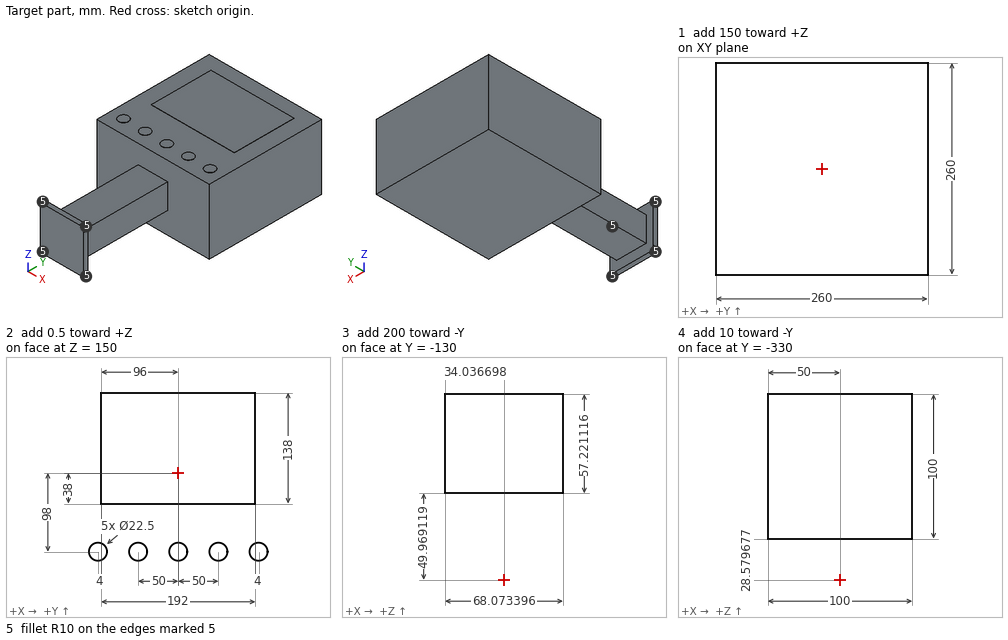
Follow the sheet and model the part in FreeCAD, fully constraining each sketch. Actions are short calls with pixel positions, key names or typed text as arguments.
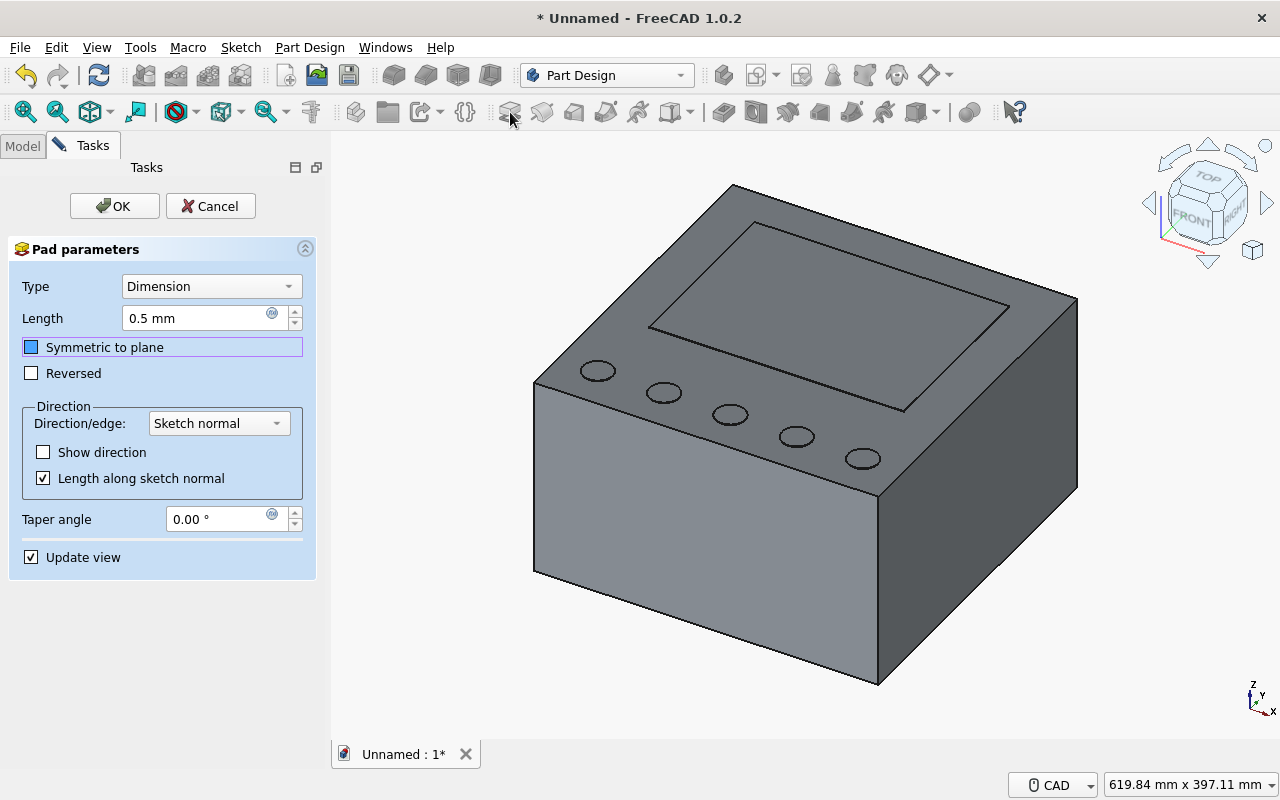
click(115, 206)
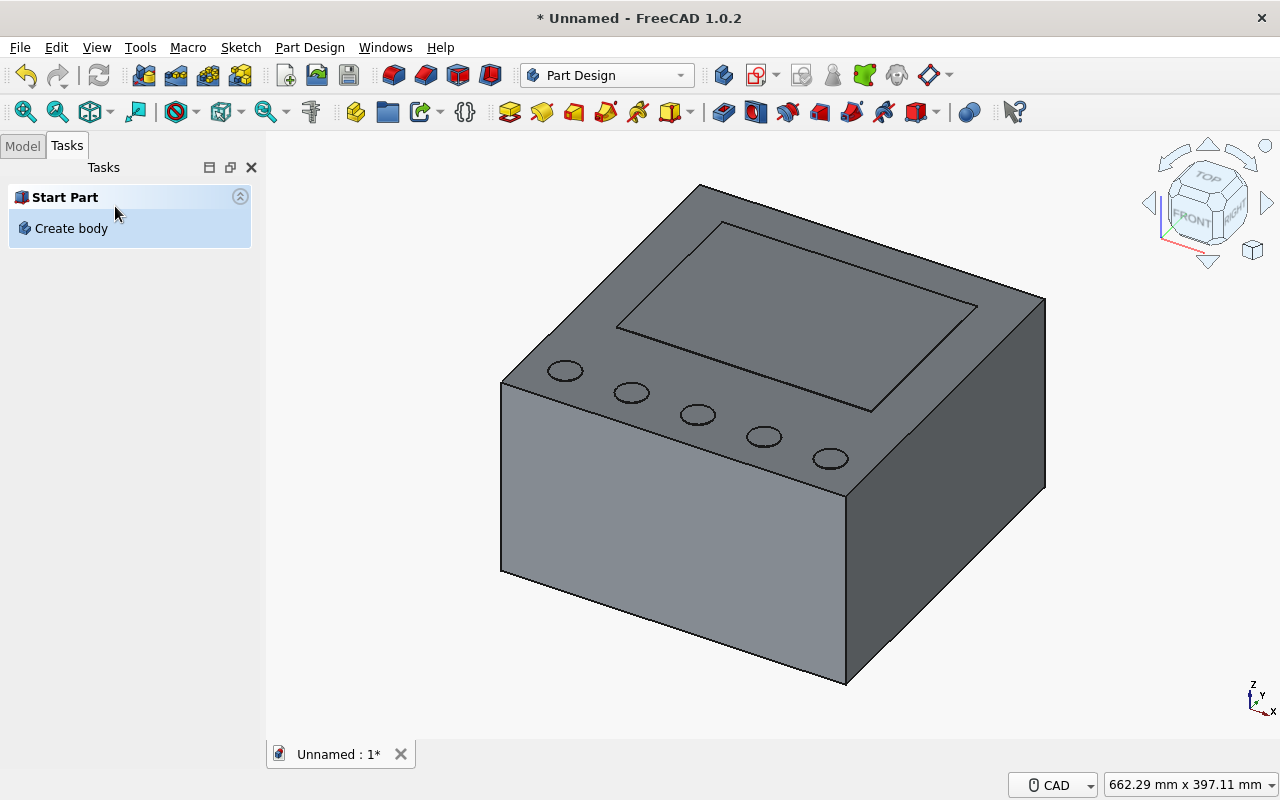
click(723, 549)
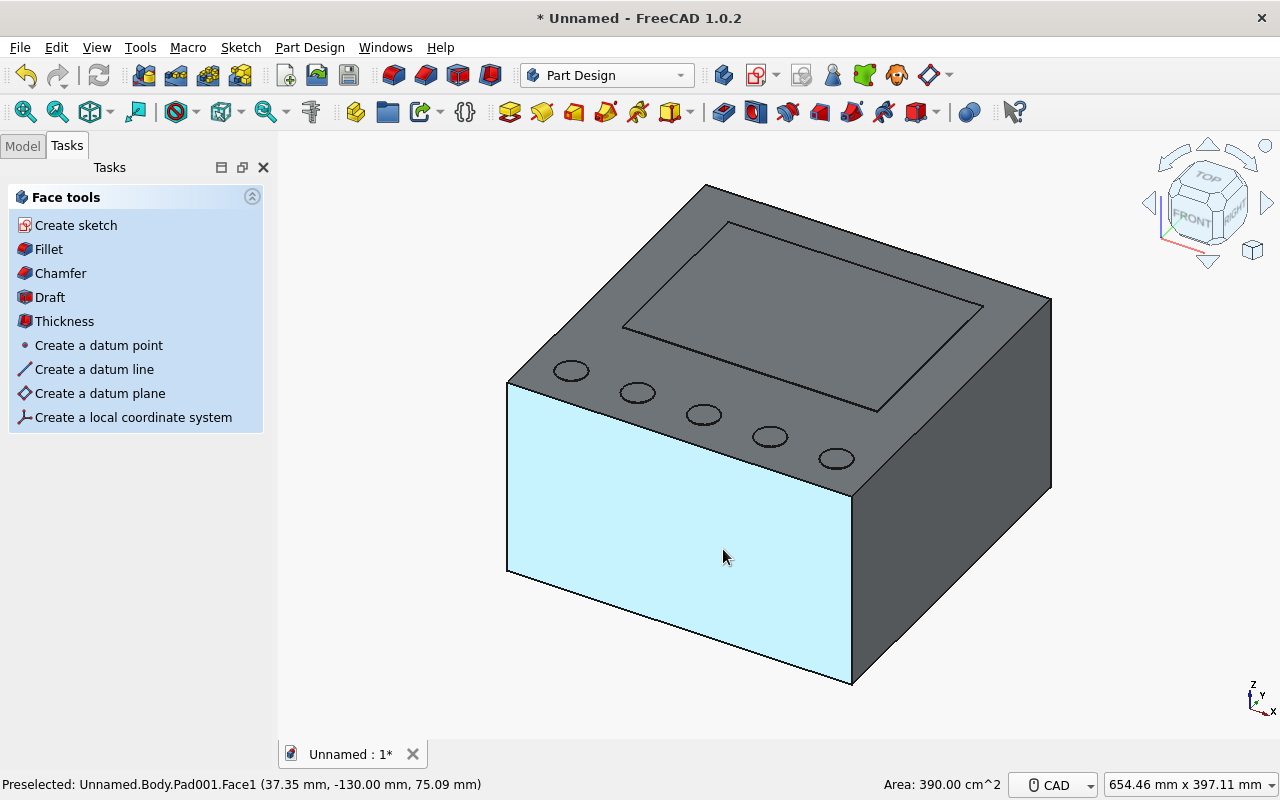
click(756, 76)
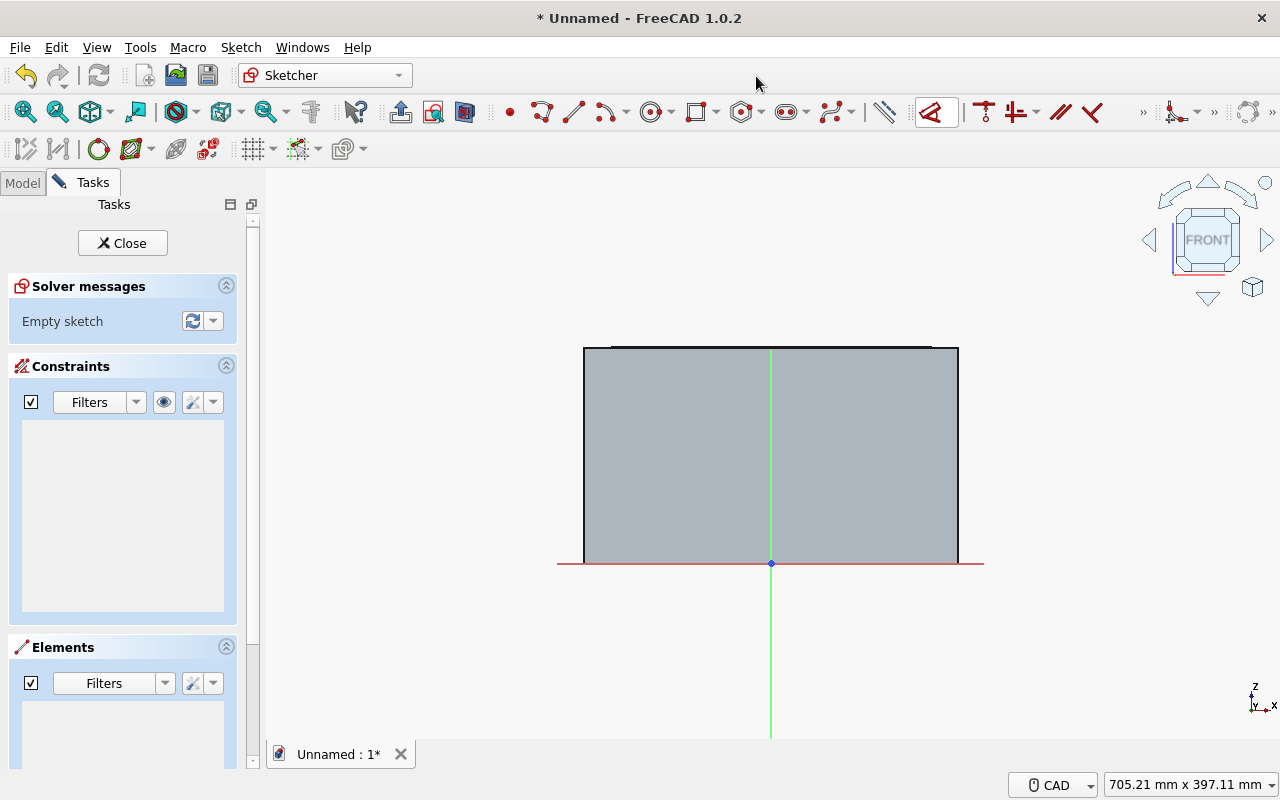
scroll(826, 513, up, 4)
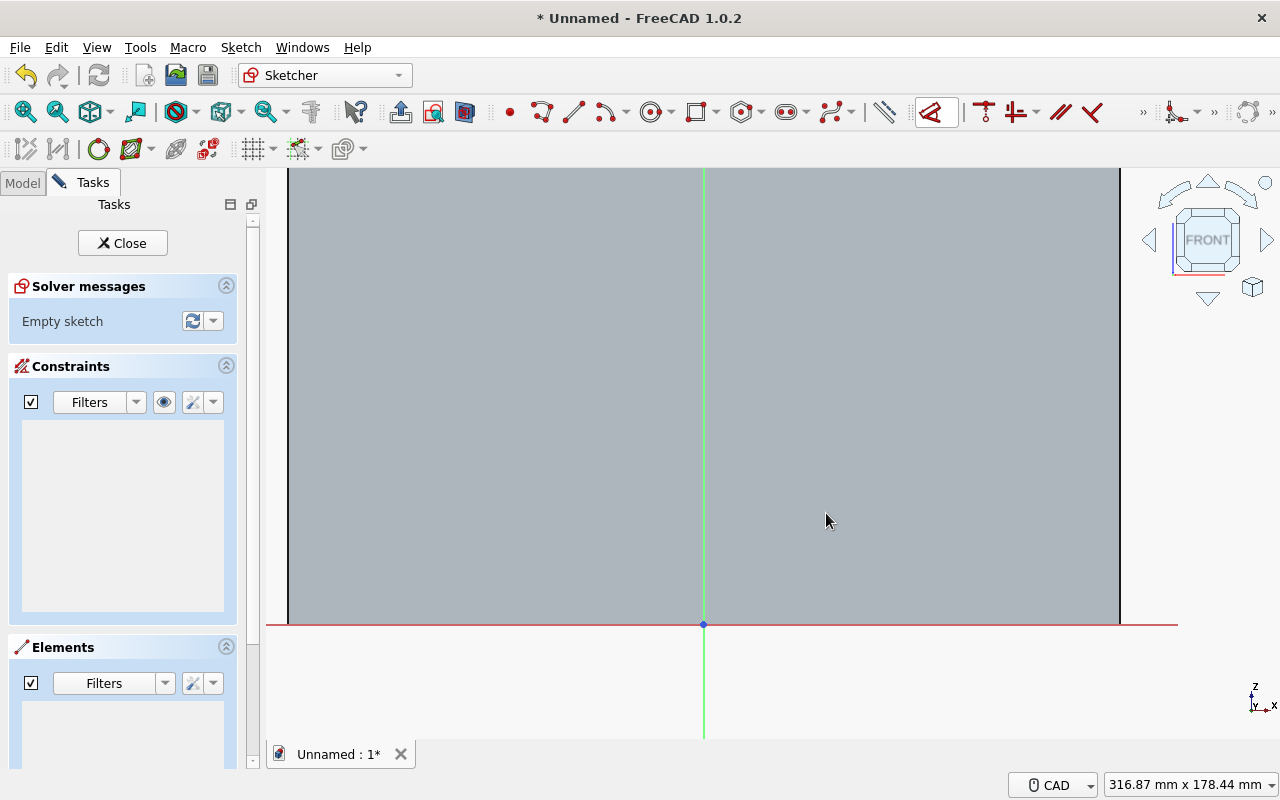
click(696, 112)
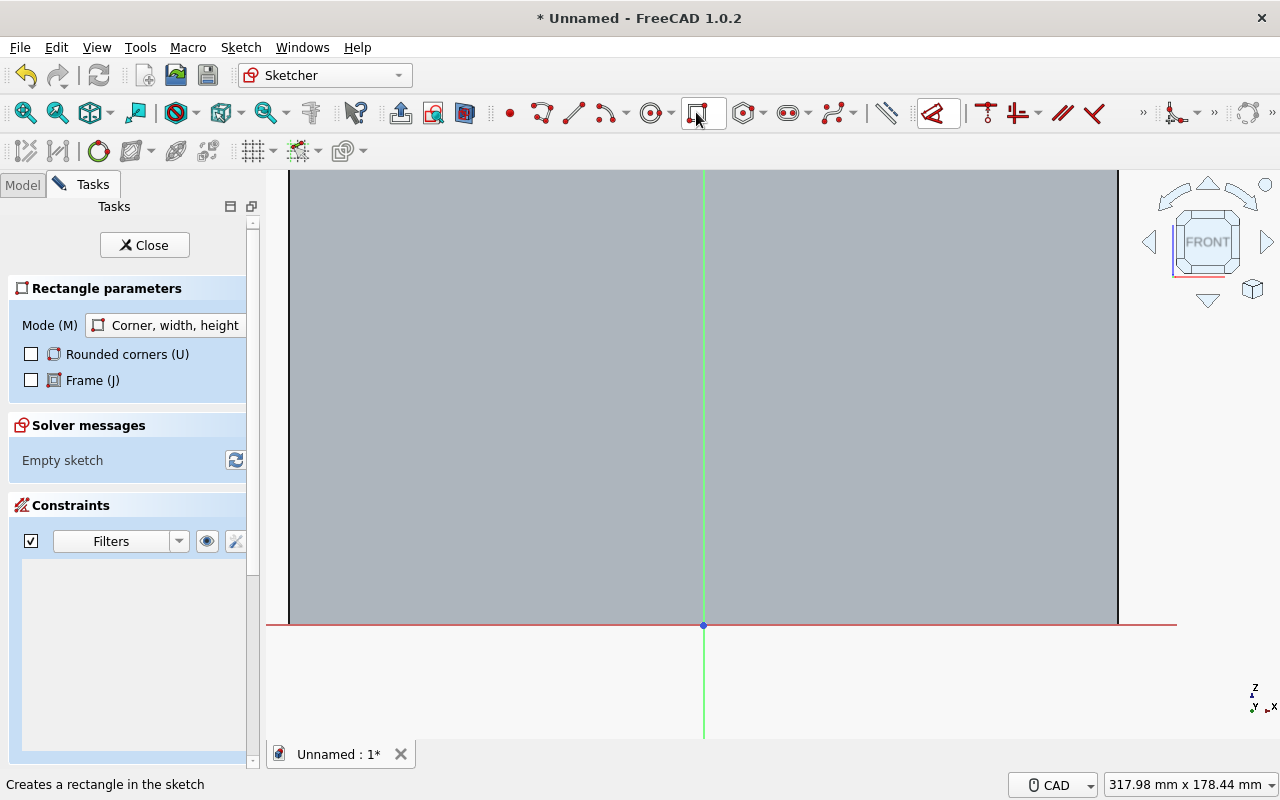
click(595, 283)
move(812, 466)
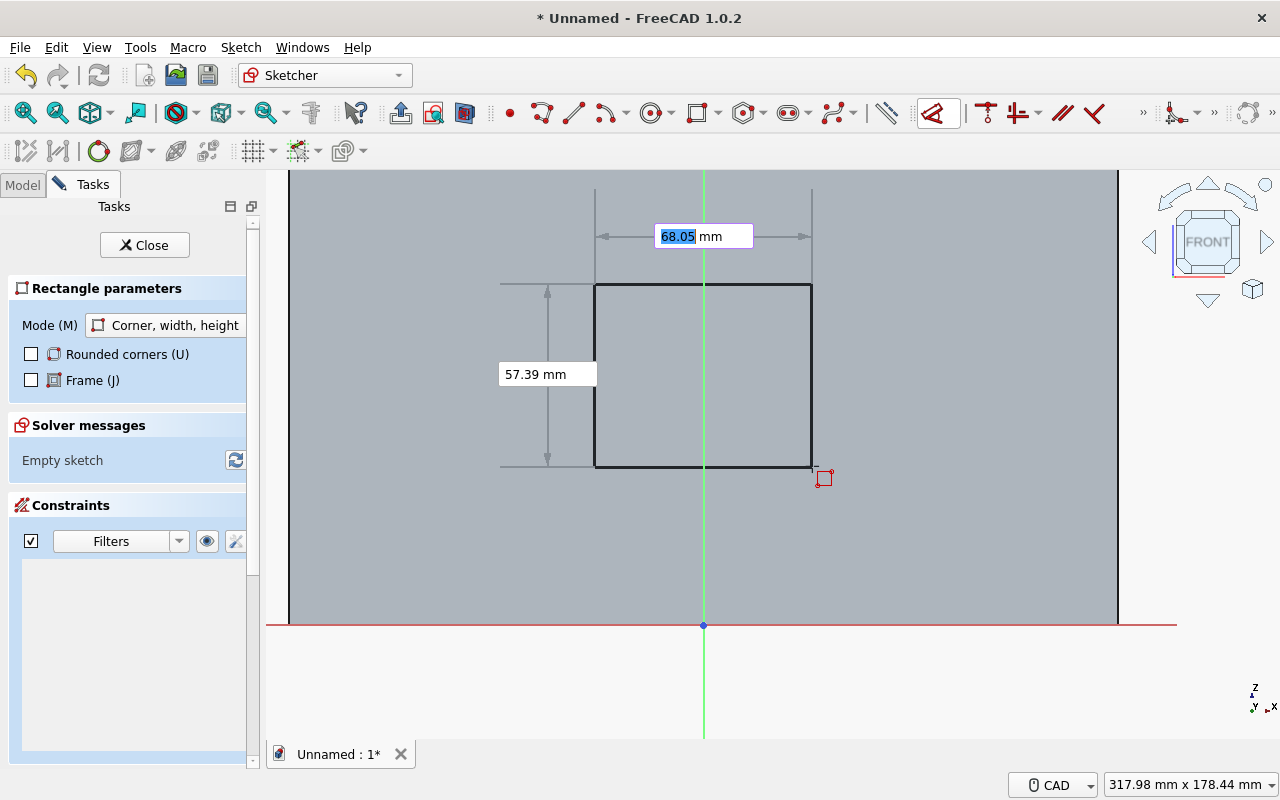
text(68.073396)
key(Tab)
text(57.221116)
key(Return)
key(Escape)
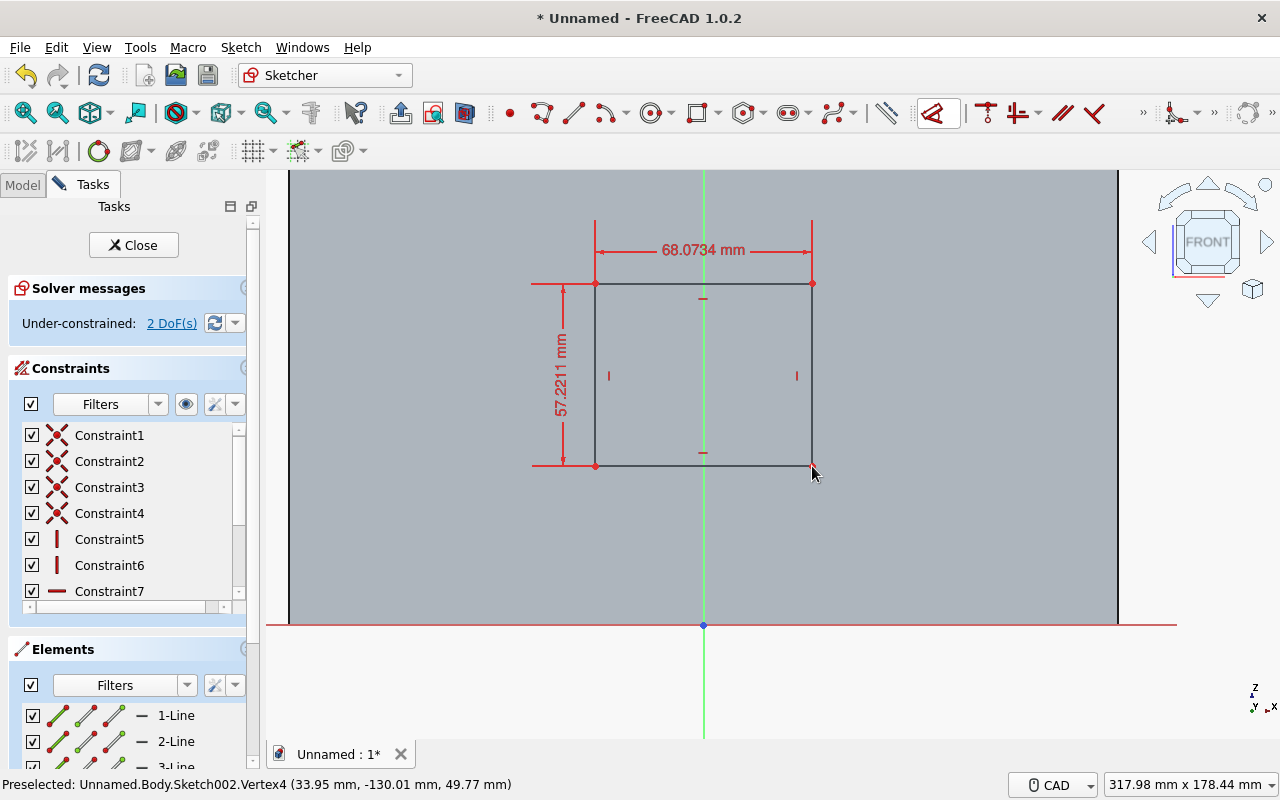
click(595, 284)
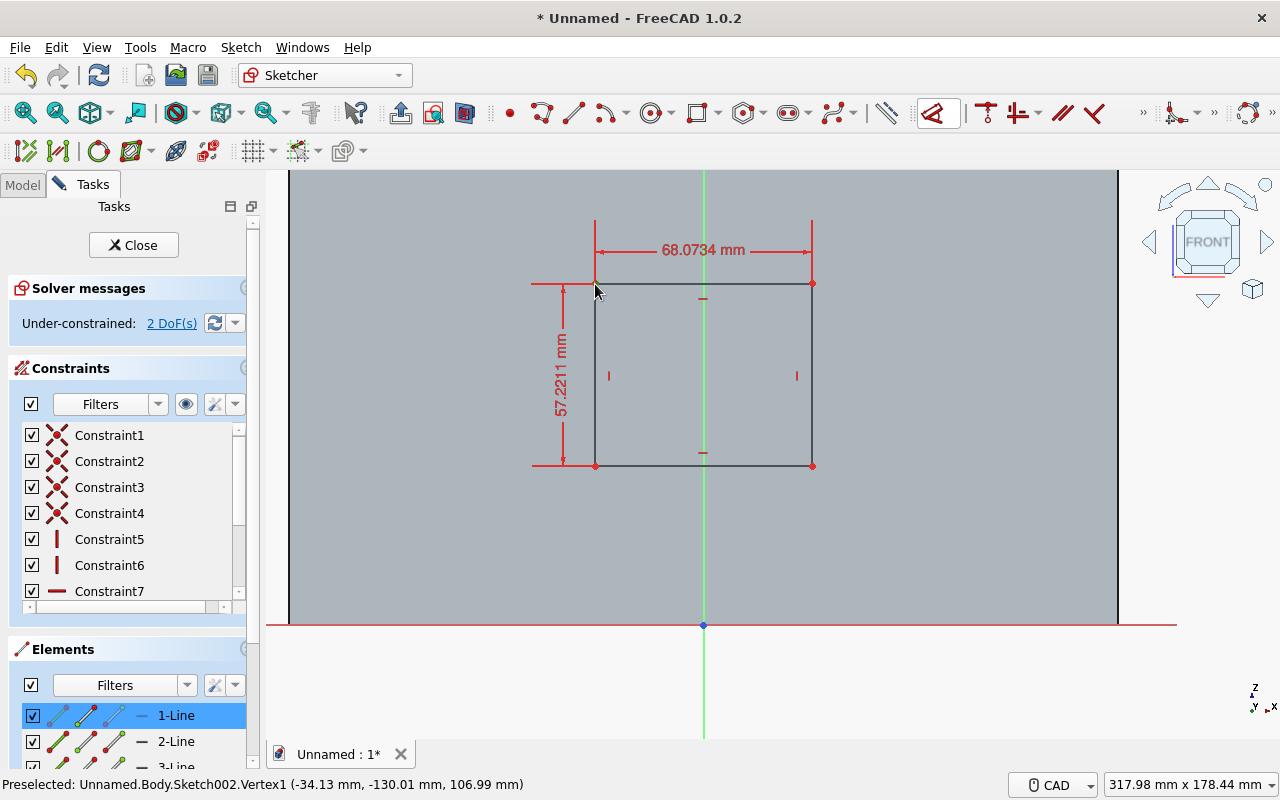
key(l)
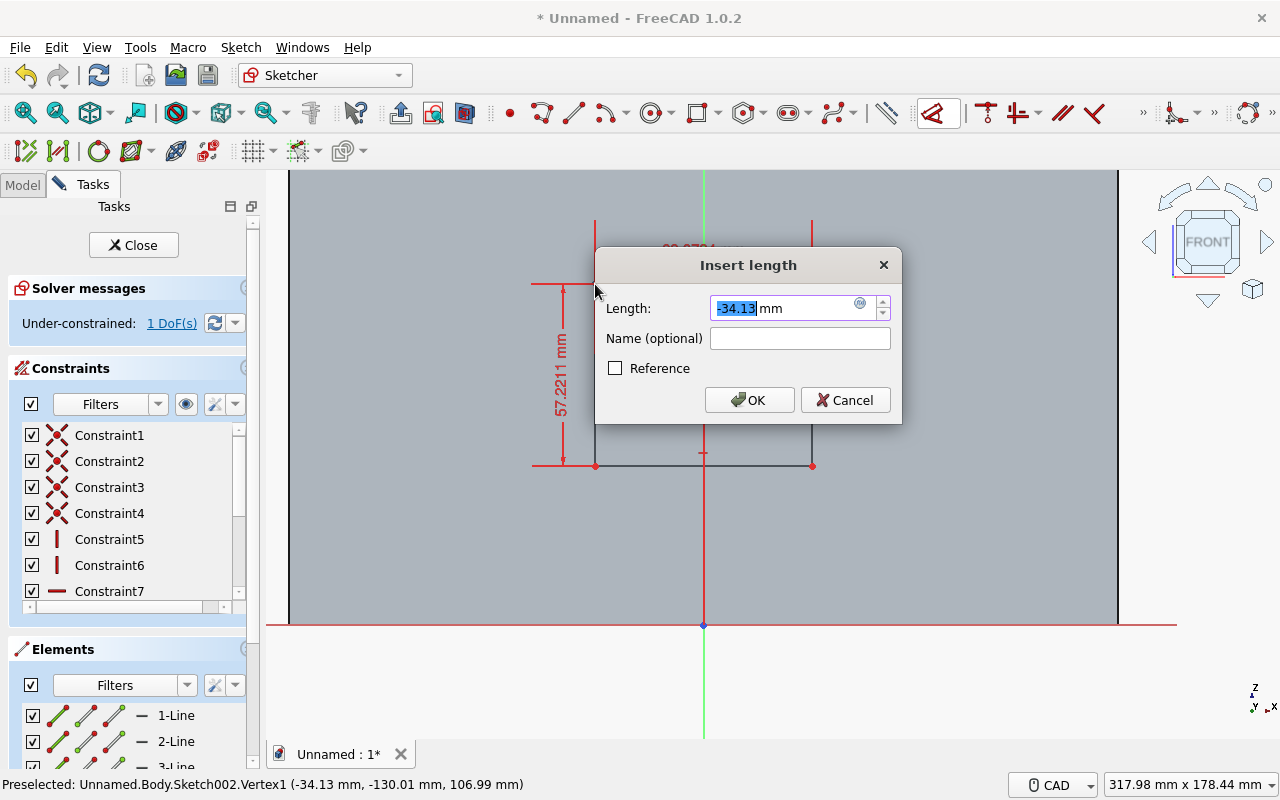
text(-34.036698)
key(Return)